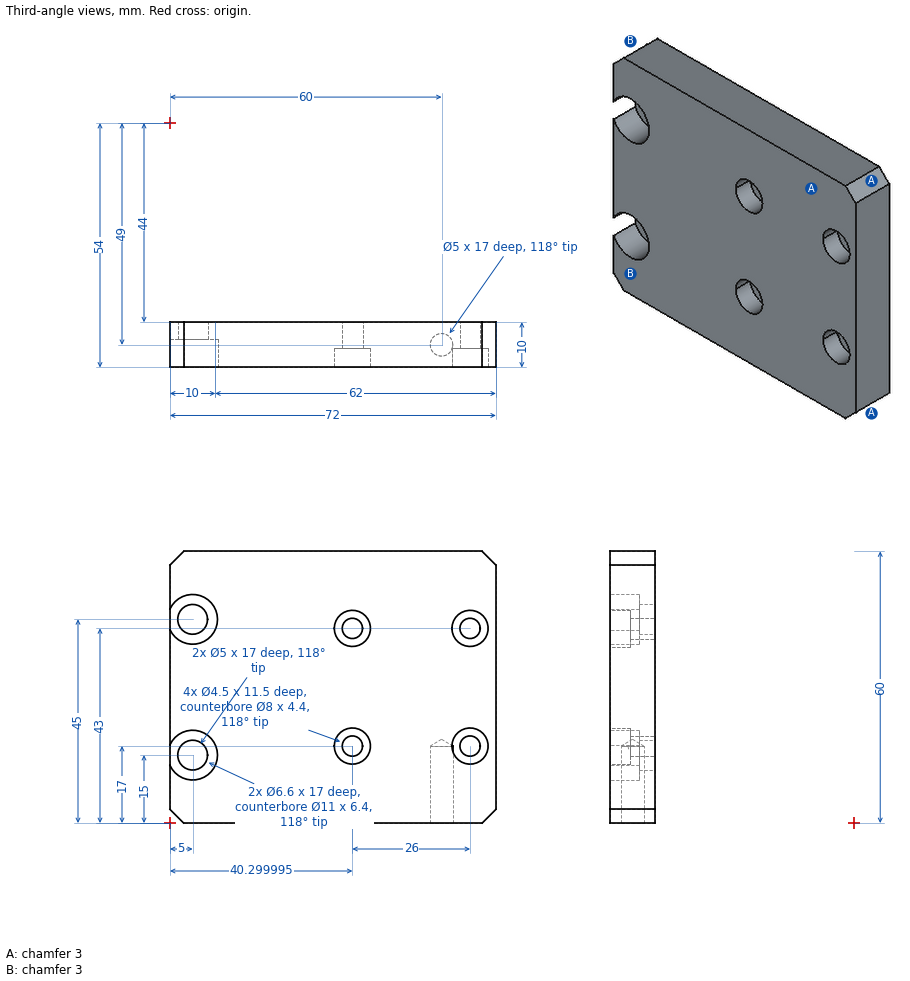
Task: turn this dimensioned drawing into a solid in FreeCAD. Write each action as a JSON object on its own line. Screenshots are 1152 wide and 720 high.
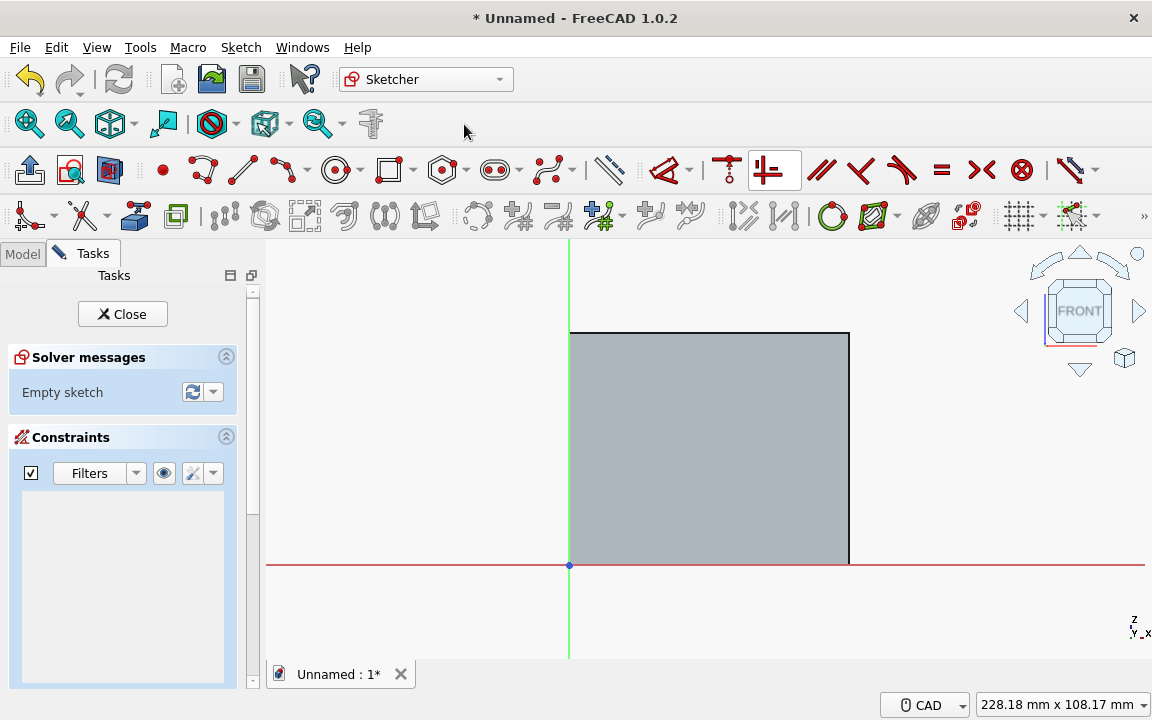
{"action": "scroll", "coordinate": [828, 536], "scroll_direction": "up", "scroll_amount": 2}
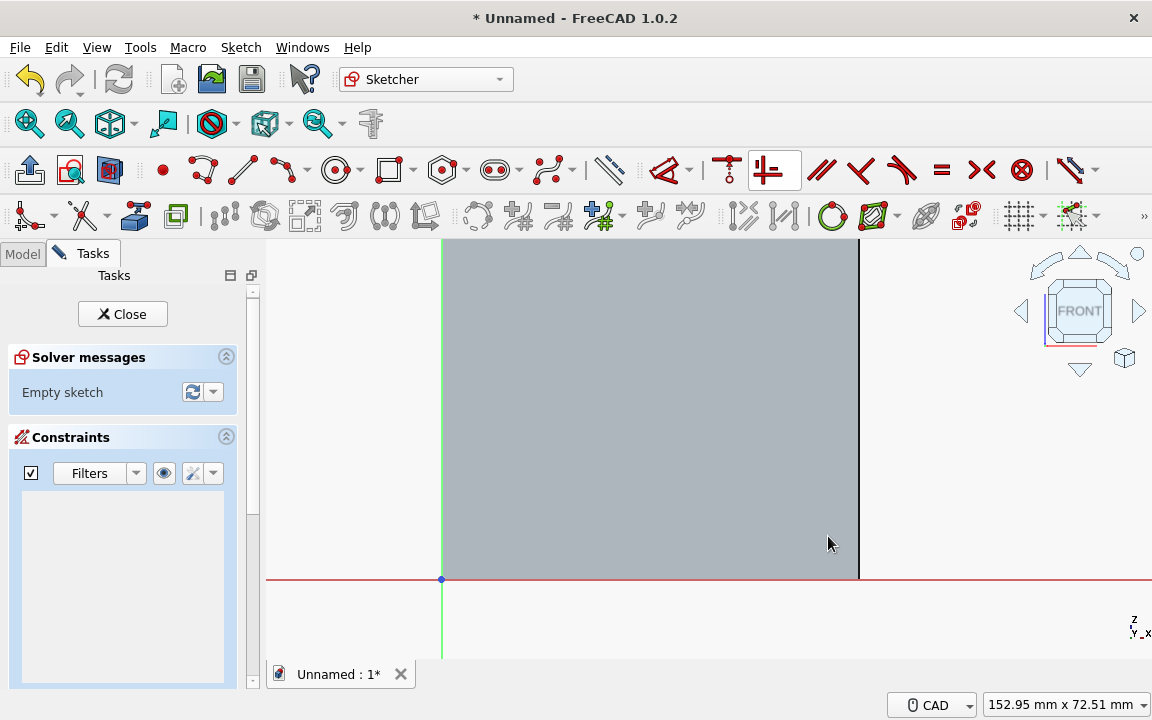
{"action": "left_click", "coordinate": [336, 170]}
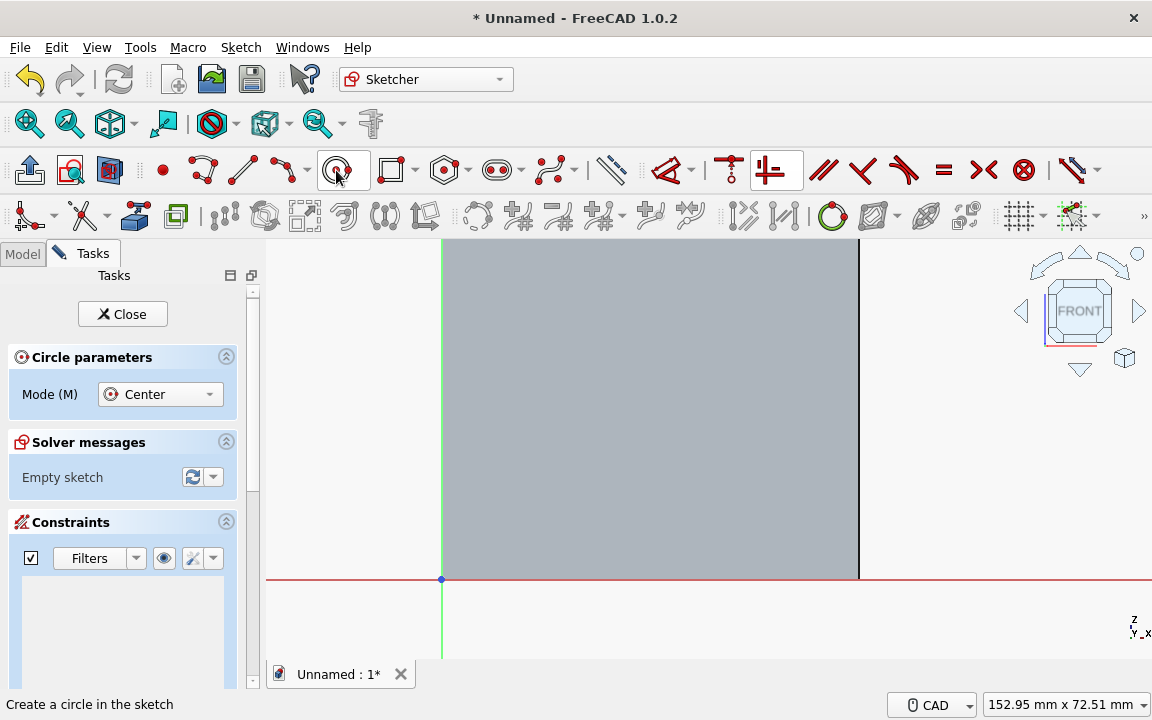
{"action": "scroll", "coordinate": [675, 481], "scroll_direction": "up", "scroll_amount": 3}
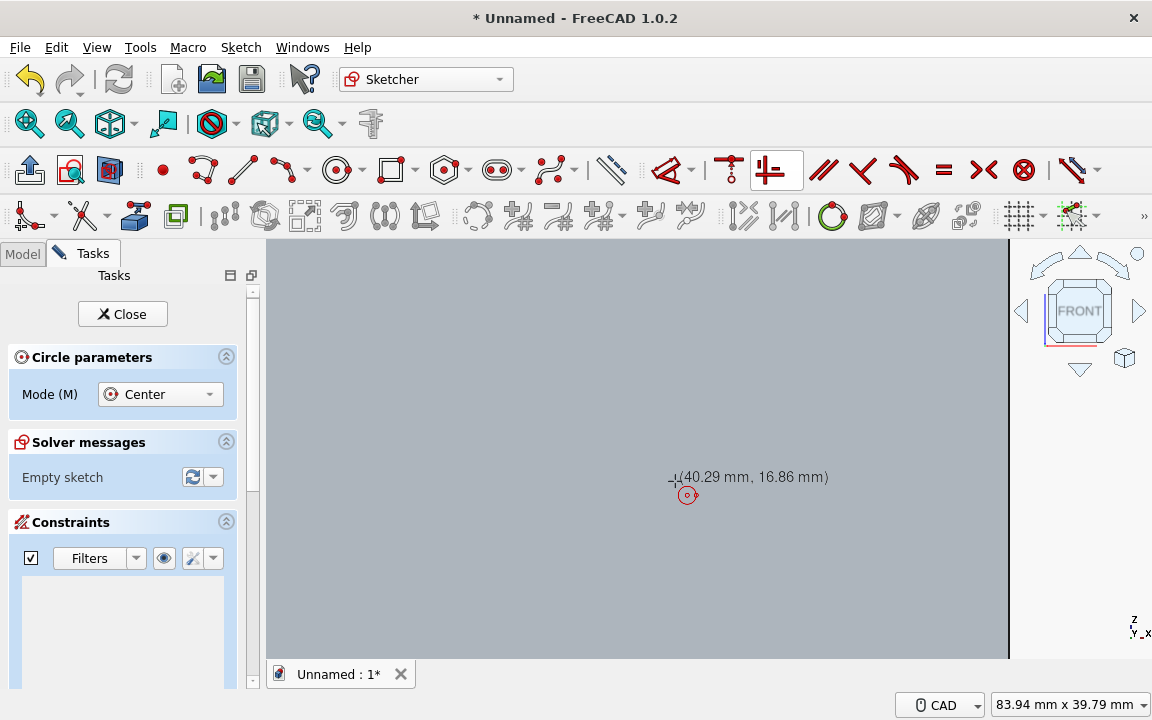
{"action": "left_click", "coordinate": [675, 481]}
{"action": "left_click", "coordinate": [692, 464]}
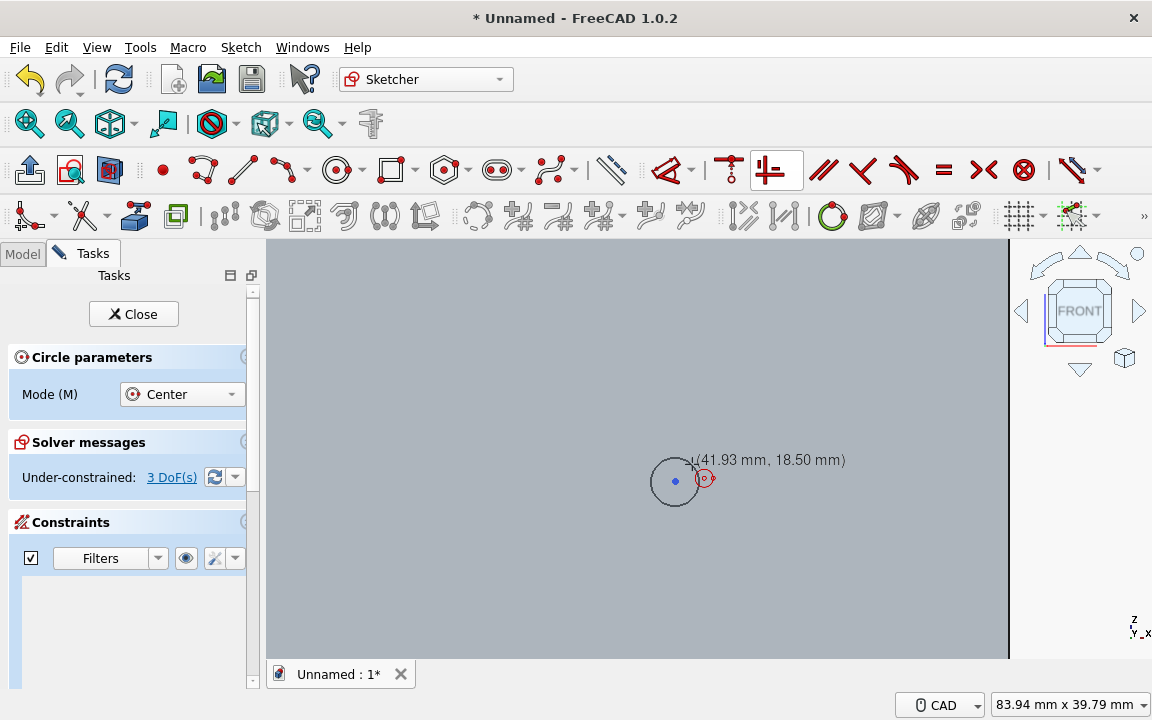
{"action": "left_click", "coordinate": [949, 481]}
{"action": "left_click", "coordinate": [966, 464]}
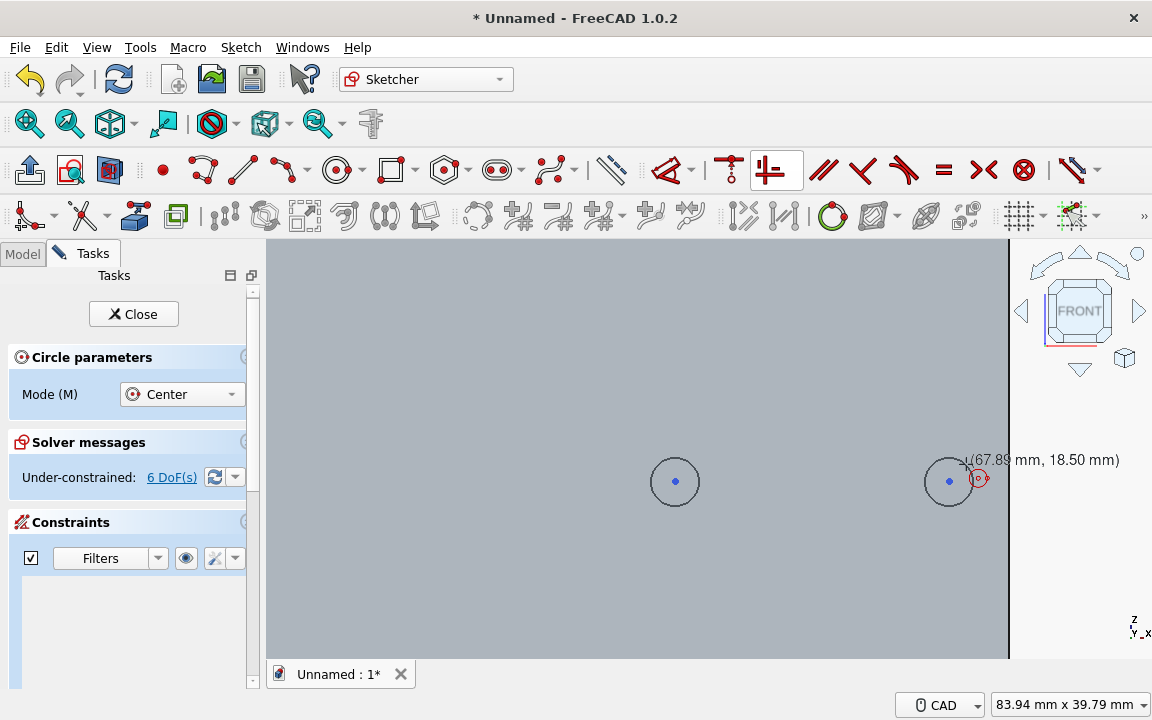
{"action": "scroll", "coordinate": [676, 483], "scroll_direction": "down", "scroll_amount": 3}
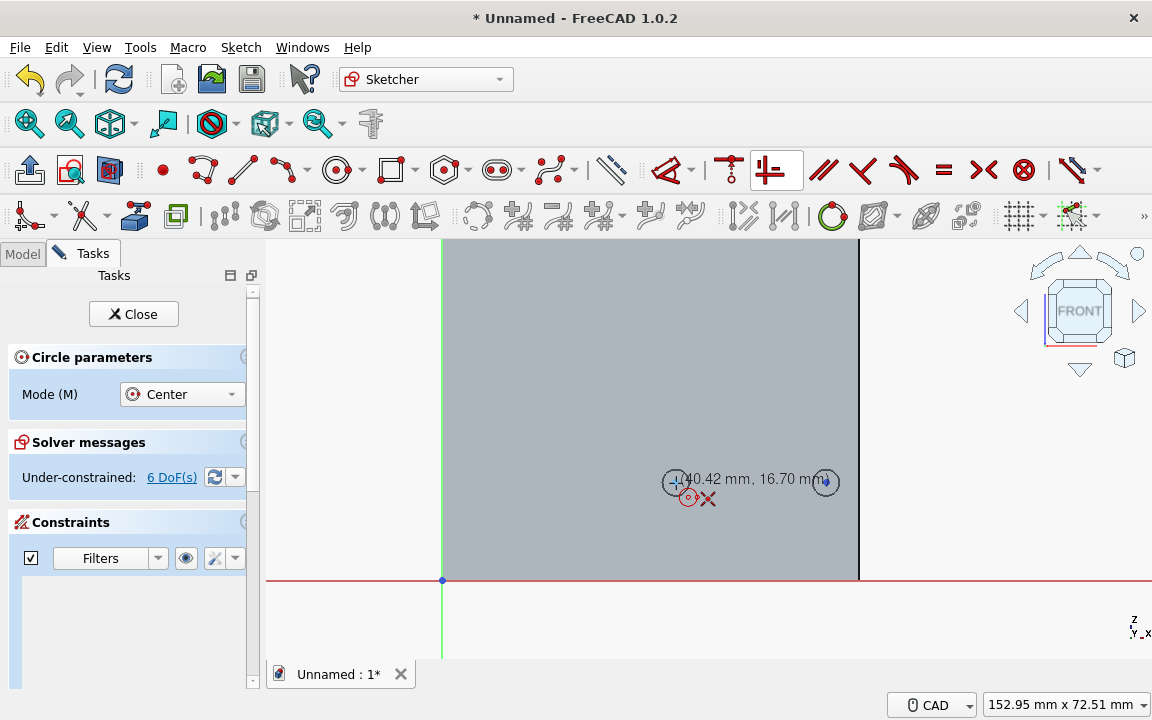
{"action": "scroll", "coordinate": [826, 331], "scroll_direction": "up", "scroll_amount": 3}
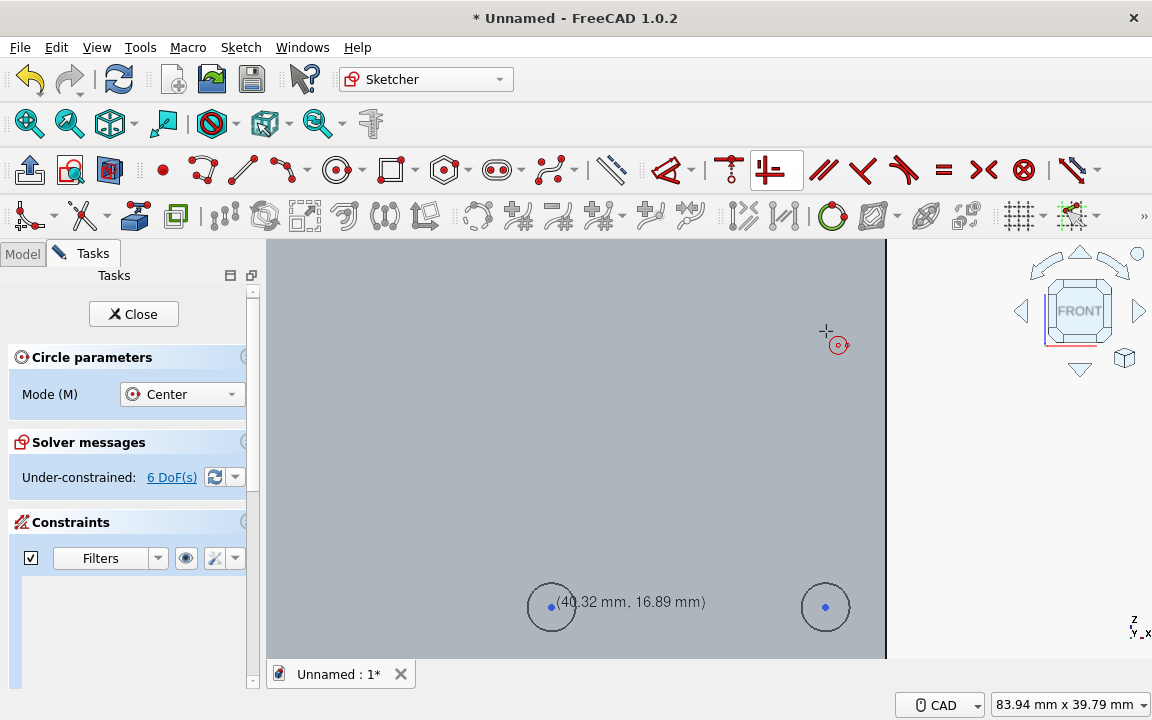
{"action": "left_click", "coordinate": [826, 332]}
{"action": "left_click", "coordinate": [843, 315]}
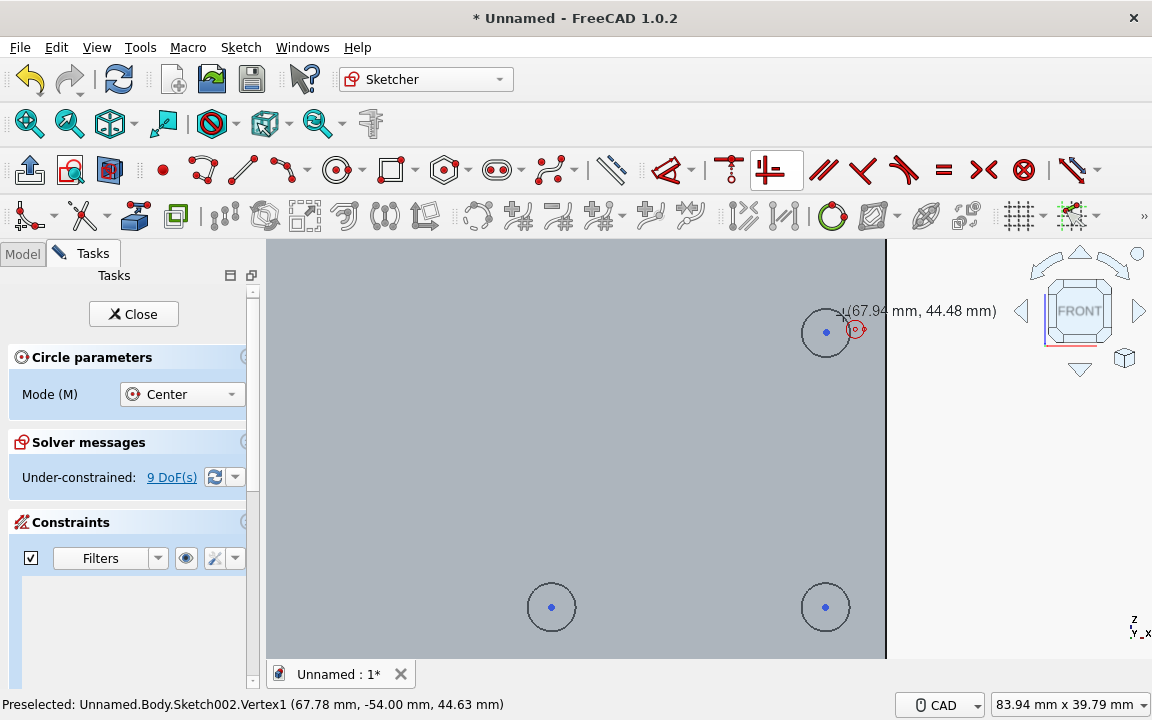
{"action": "left_click", "coordinate": [551, 332]}
{"action": "left_click", "coordinate": [568, 315]}
{"action": "key", "text": "Escape"}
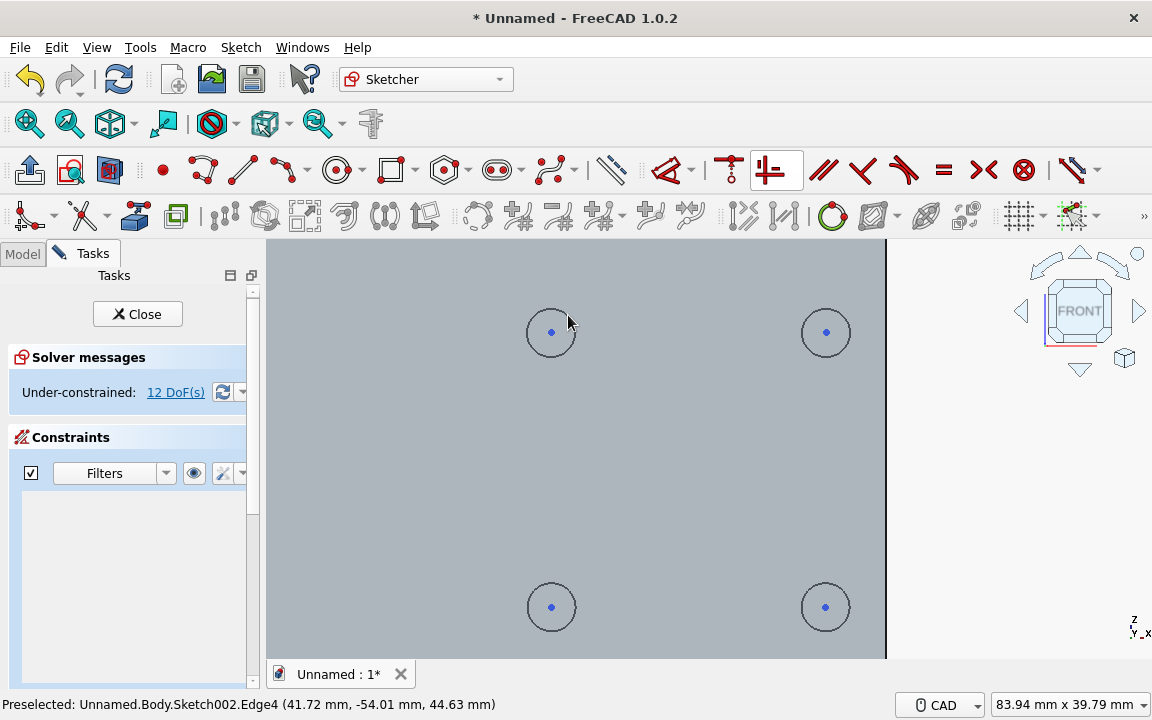
{"action": "left_click", "coordinate": [568, 590]}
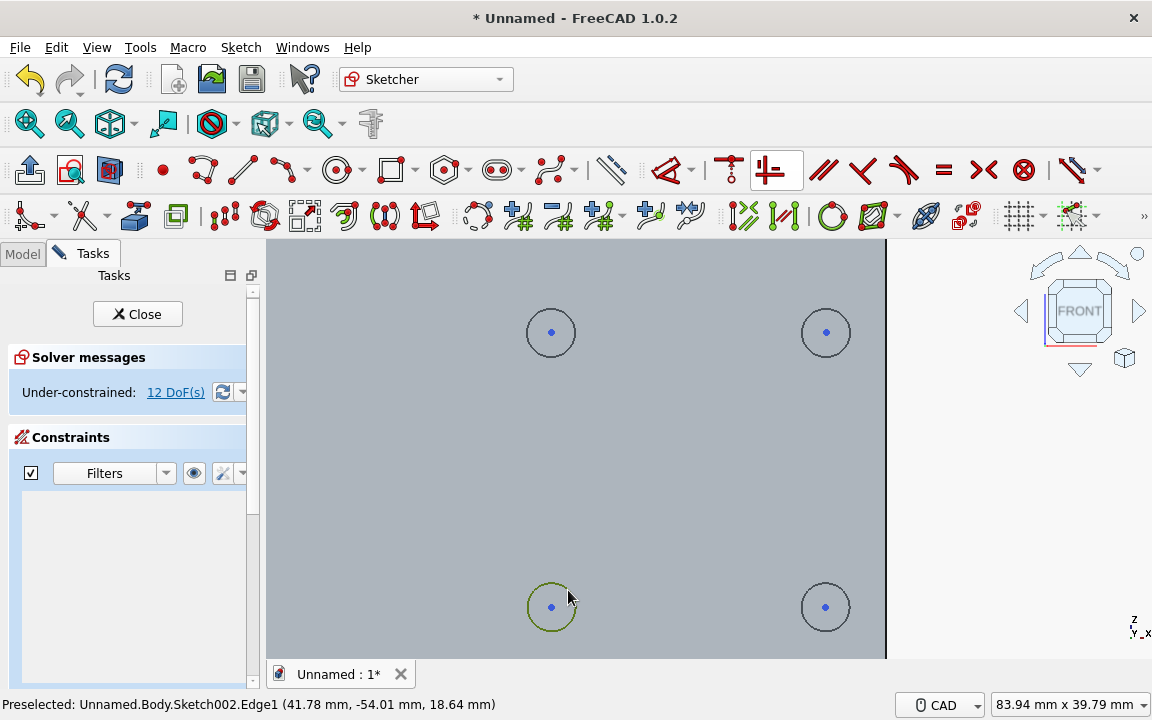
{"action": "left_click", "coordinate": [842, 590]}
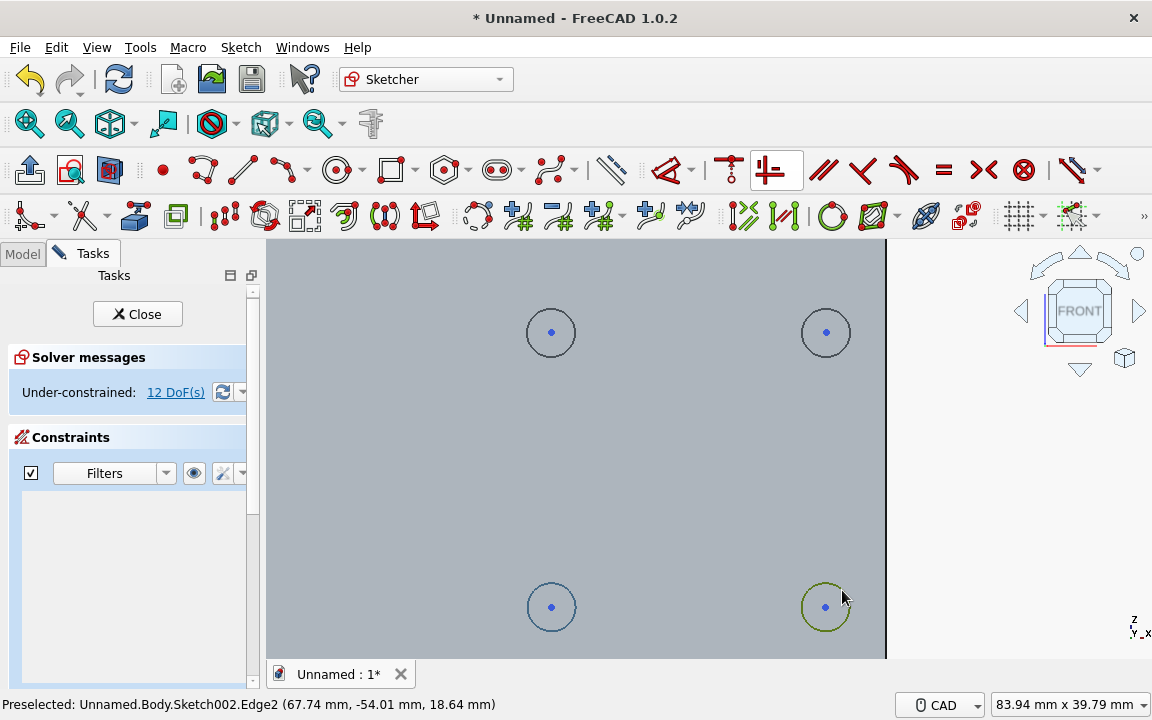
{"action": "left_click", "coordinate": [843, 316]}